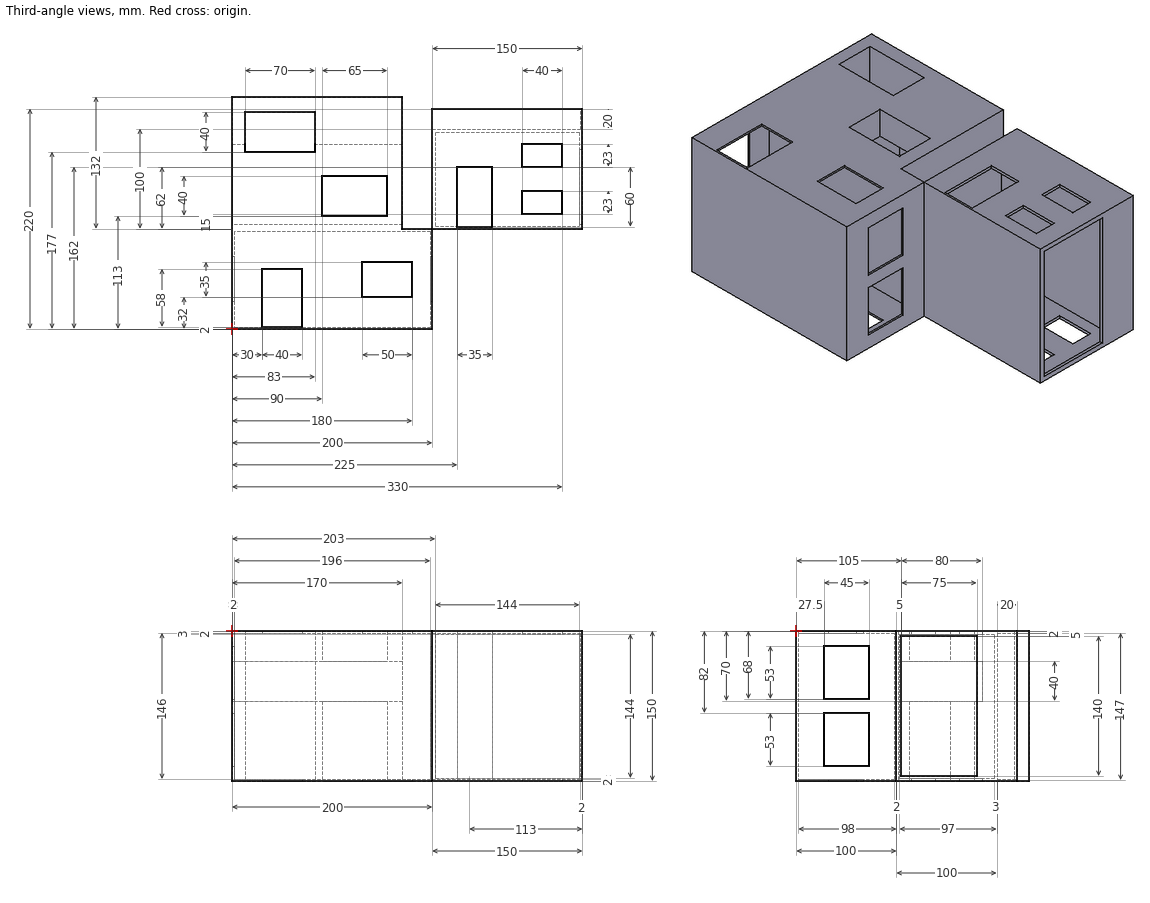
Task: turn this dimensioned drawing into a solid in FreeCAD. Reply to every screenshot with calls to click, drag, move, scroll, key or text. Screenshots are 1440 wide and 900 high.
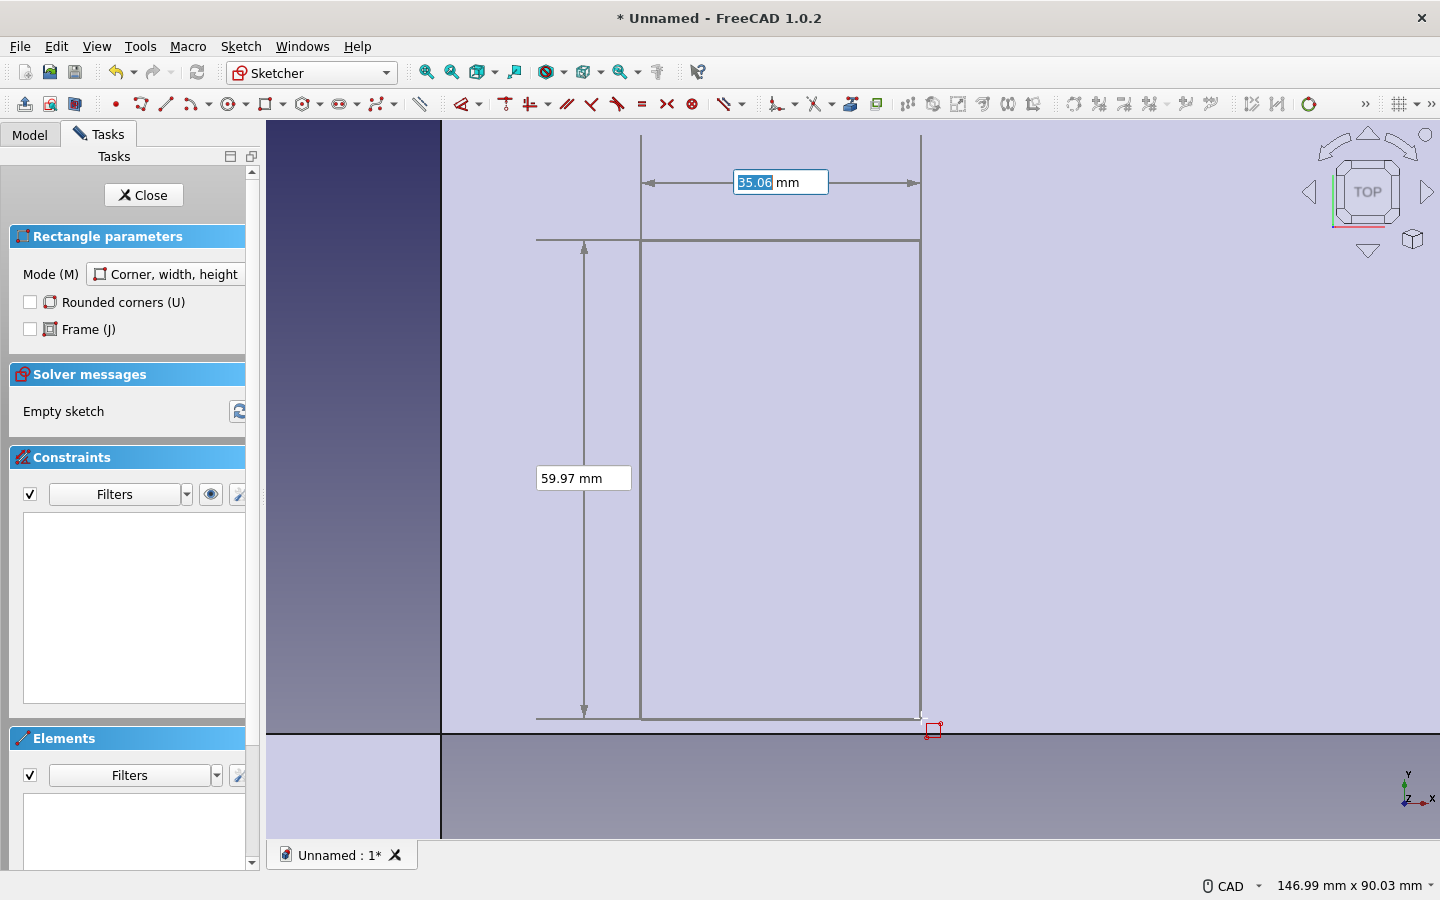
text(35)
key(Tab)
text(60)
key(Return)
key(Escape)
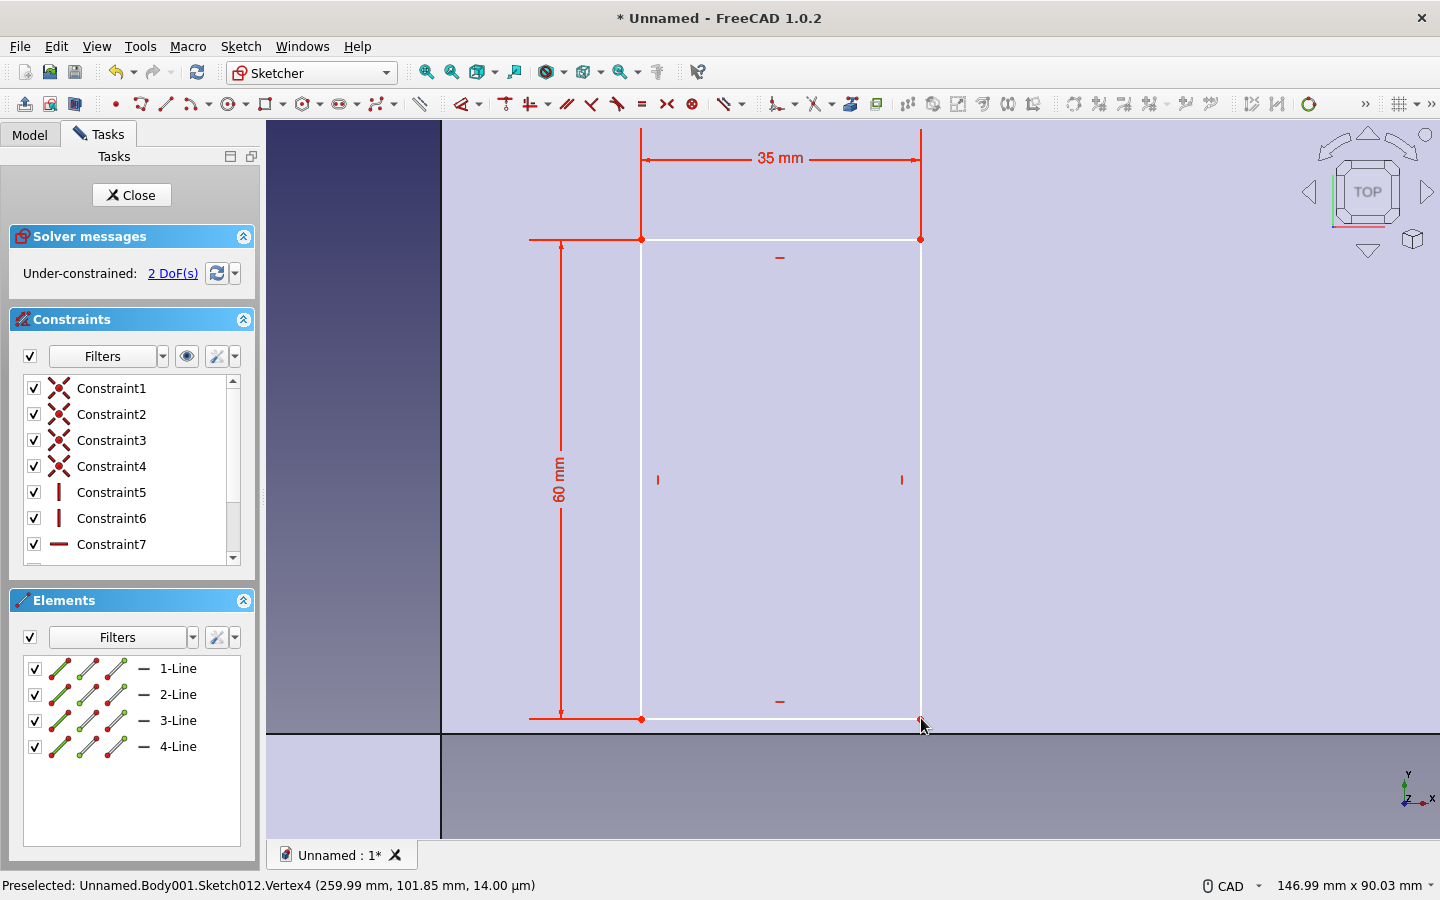
click(460, 104)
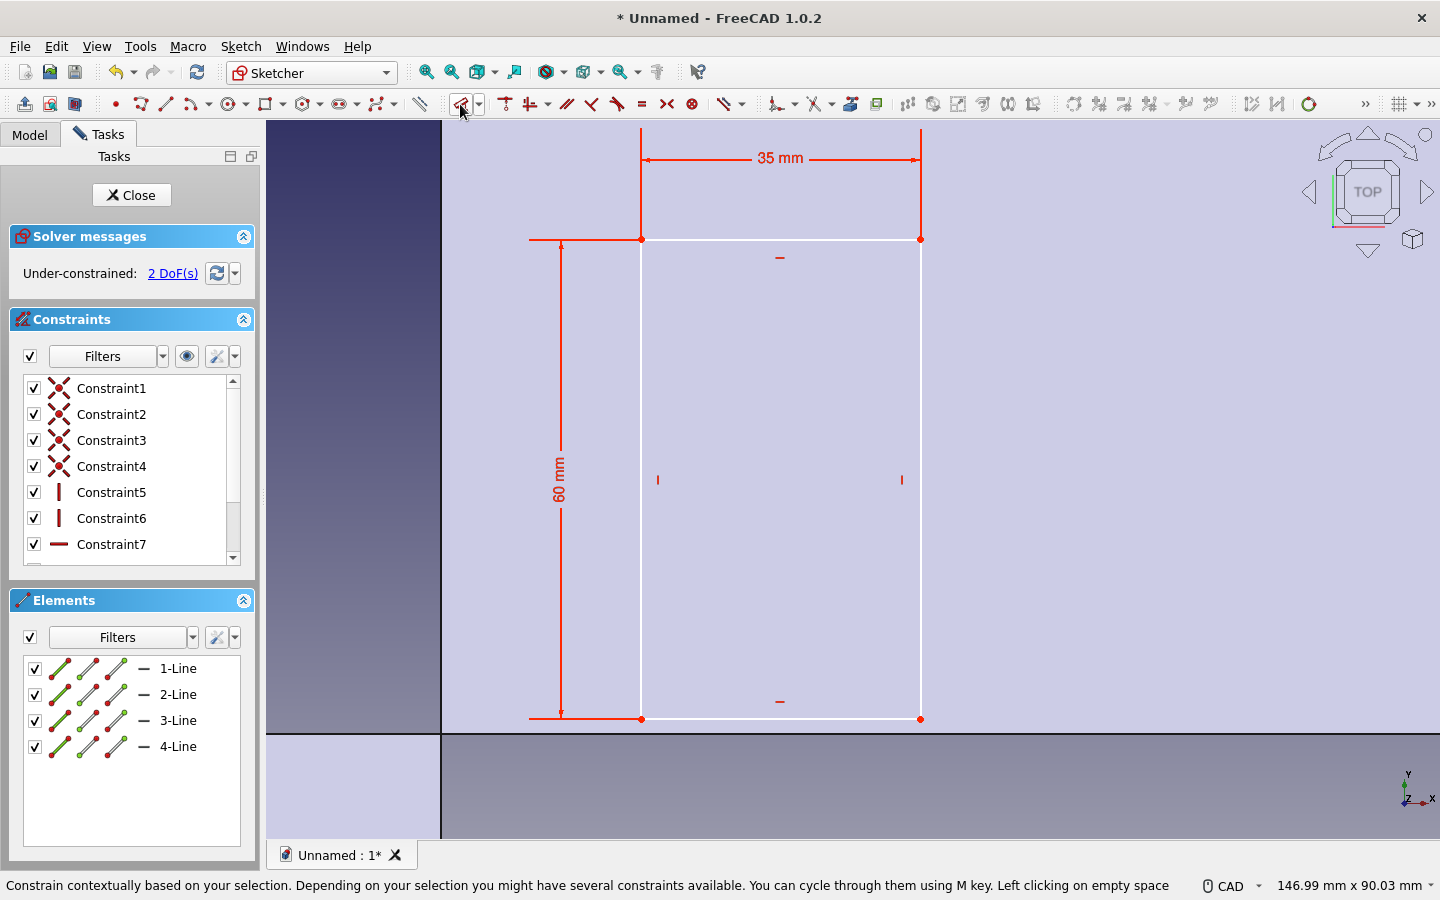
click(641, 240)
click(468, 206)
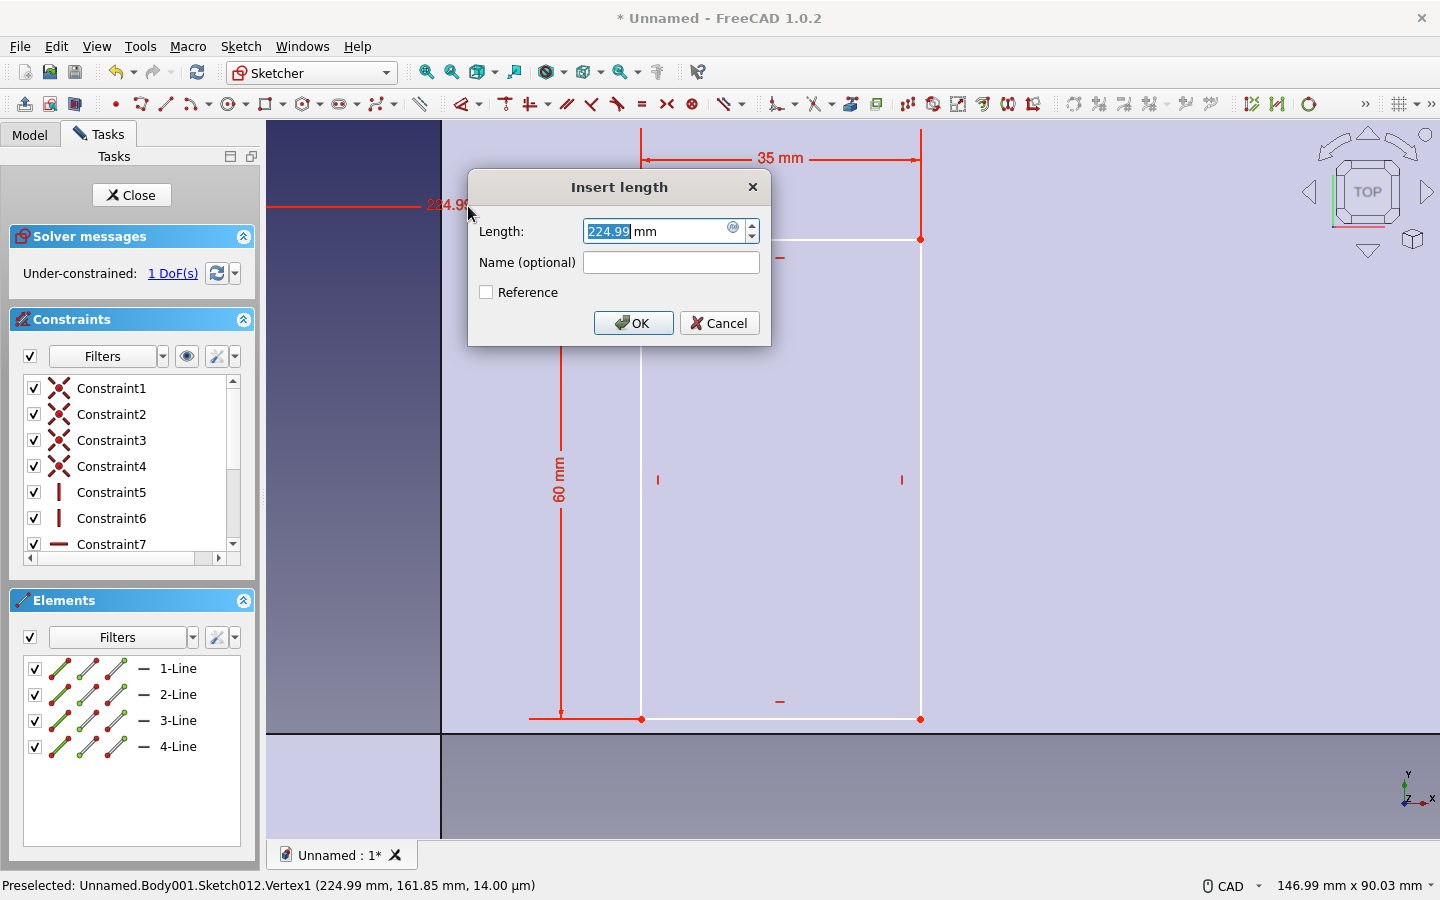
text(225)
key(Return)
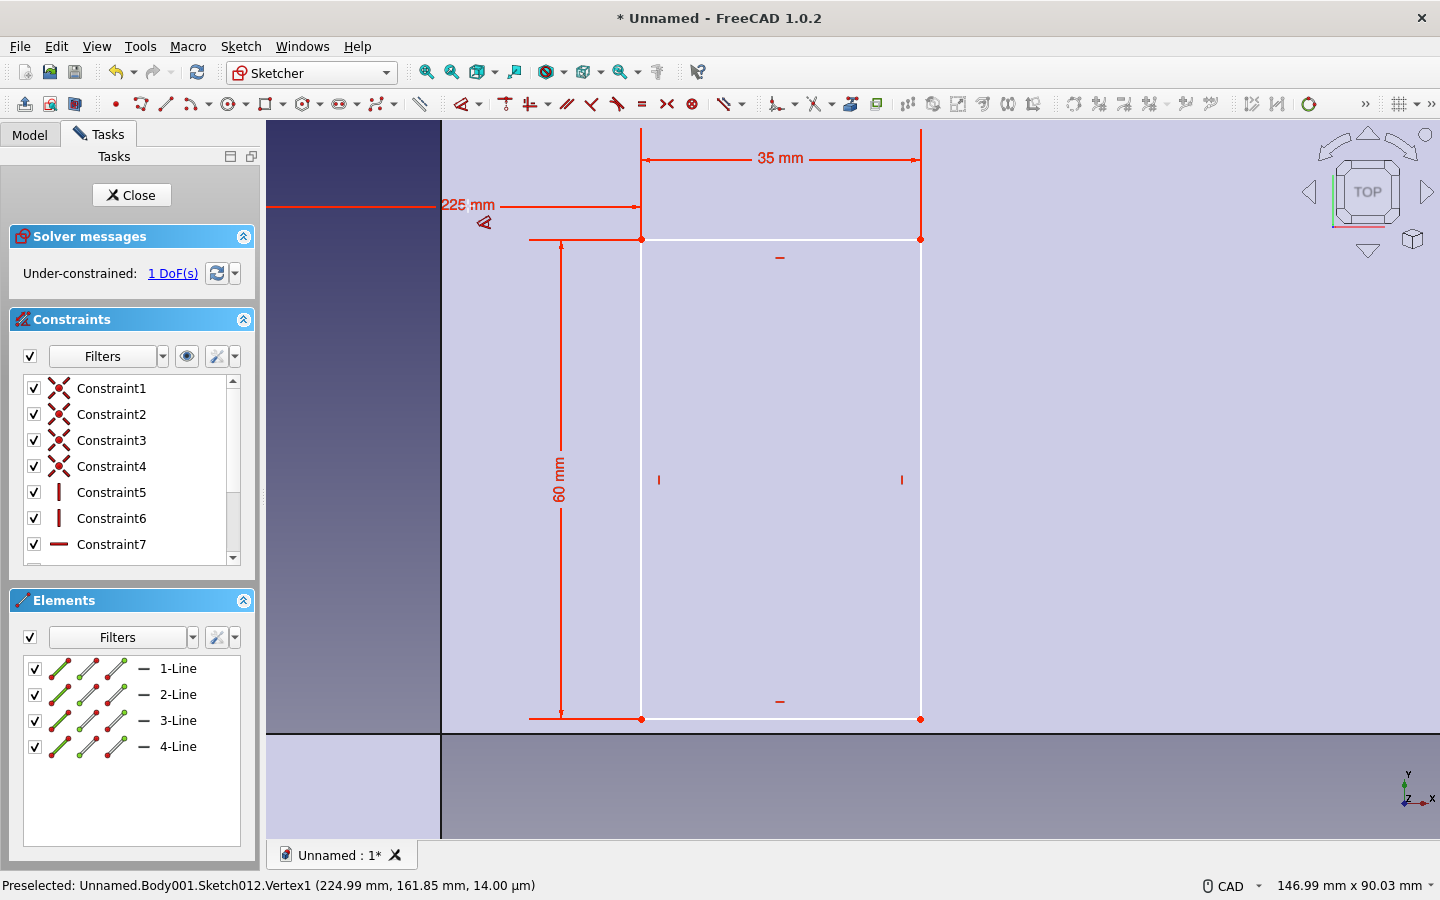
click(641, 240)
click(675, 526)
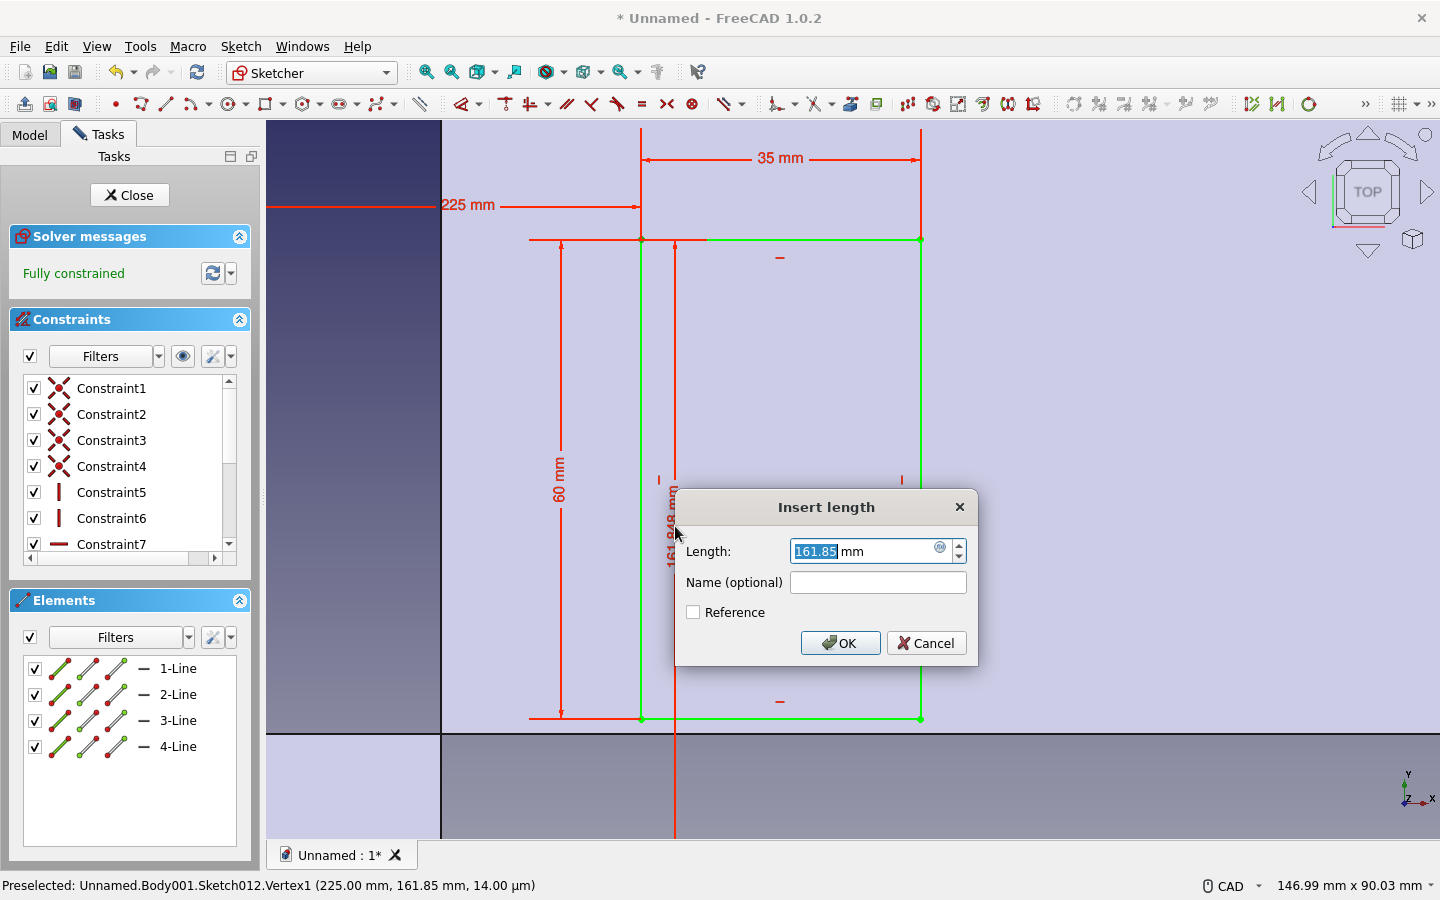
text(162)
key(Return)
key(Escape)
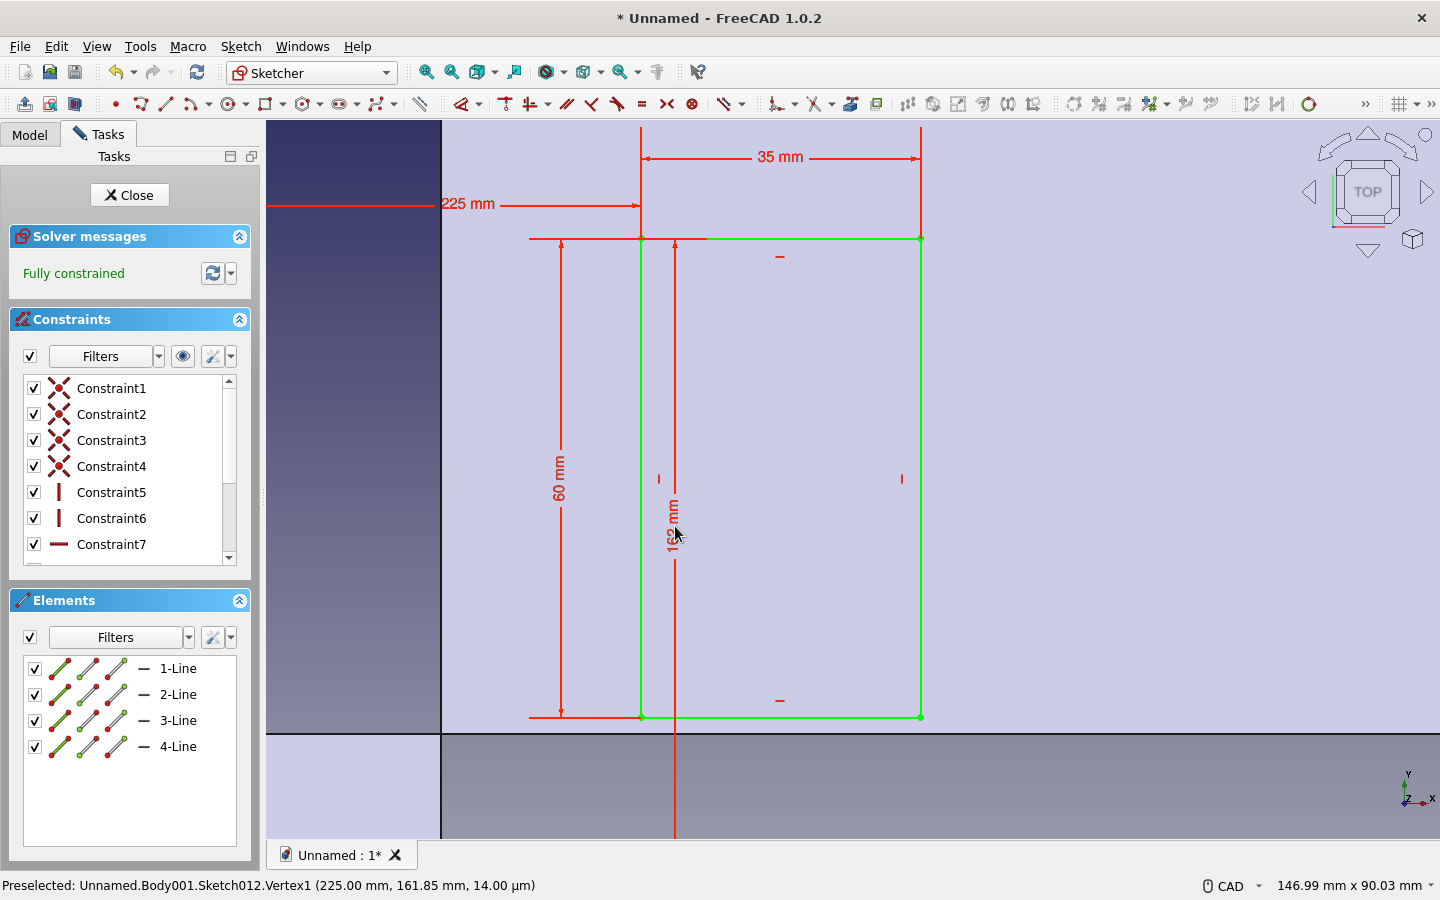
click(130, 195)